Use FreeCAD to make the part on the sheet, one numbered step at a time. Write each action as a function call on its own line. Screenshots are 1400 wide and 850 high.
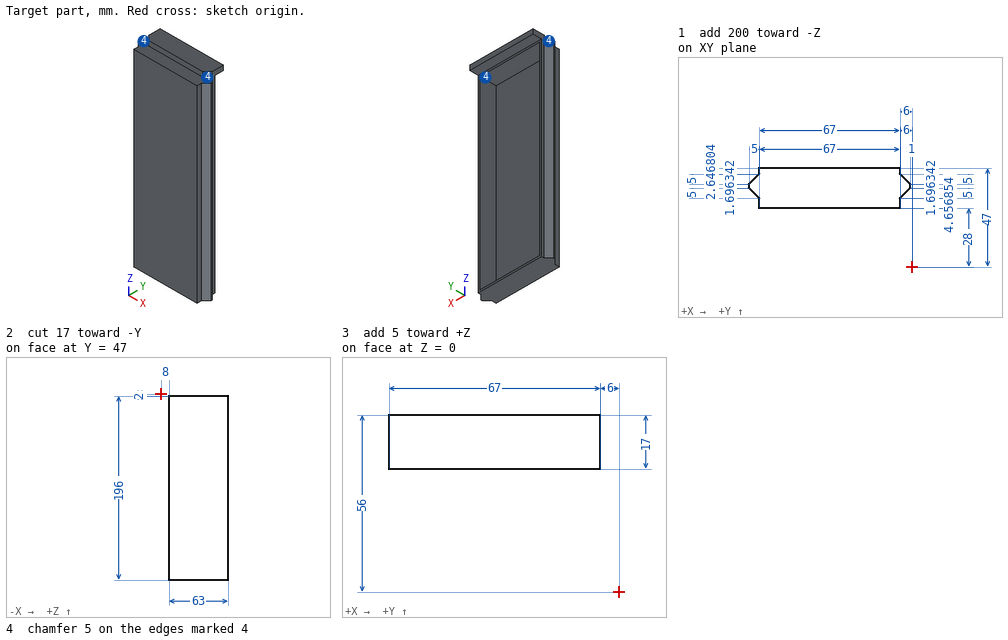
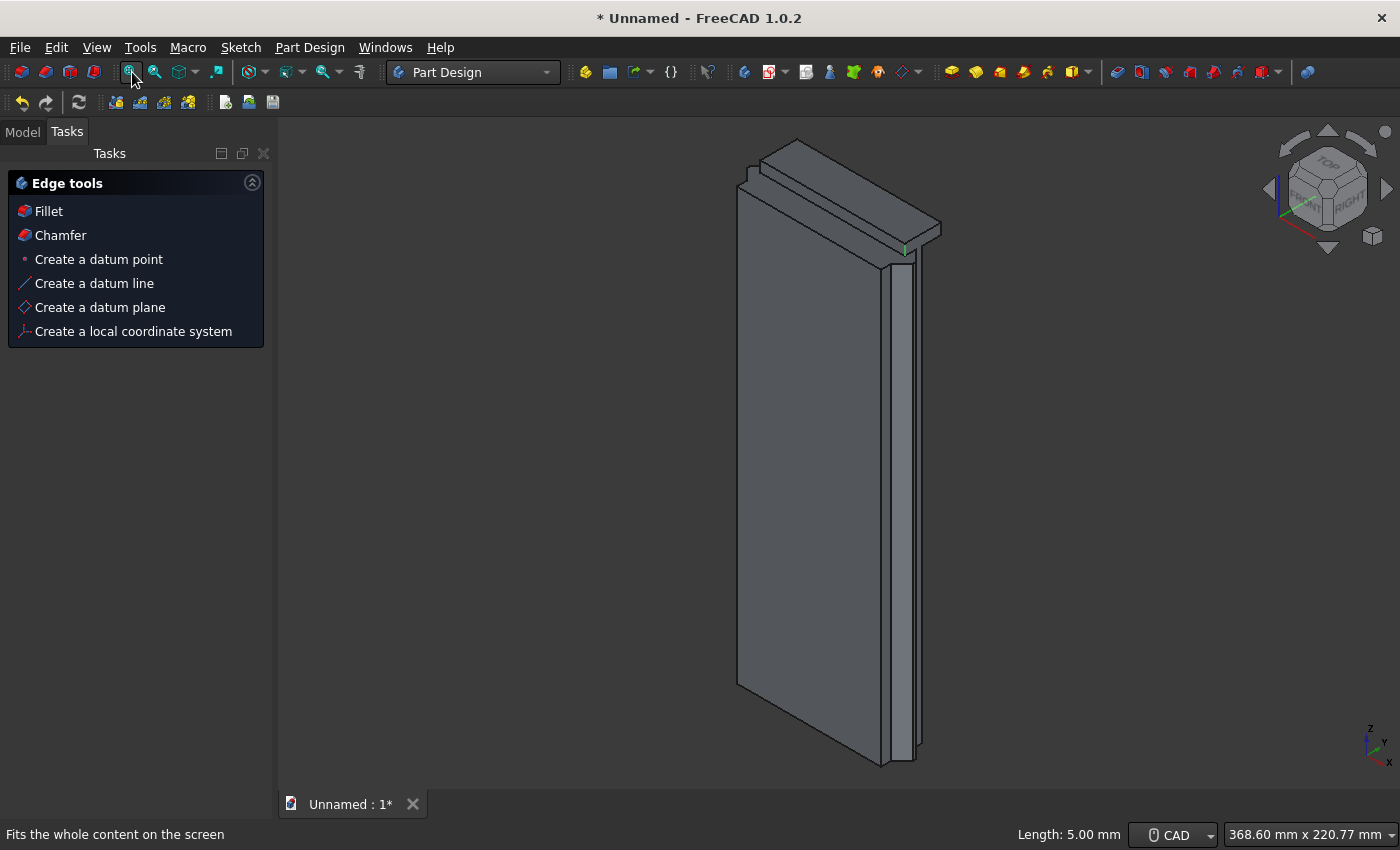
scroll(760, 166, up, 5)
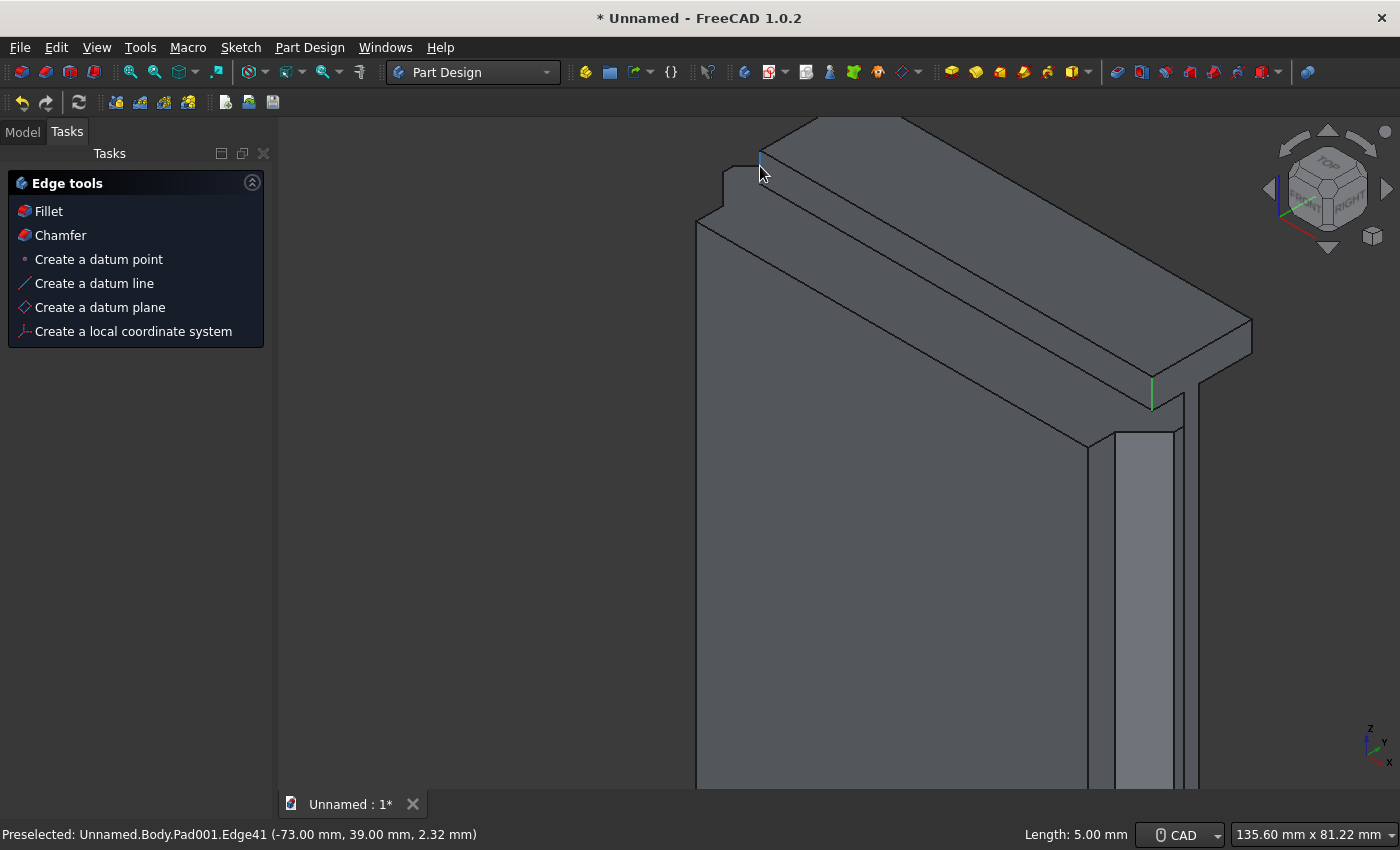
click(132, 72)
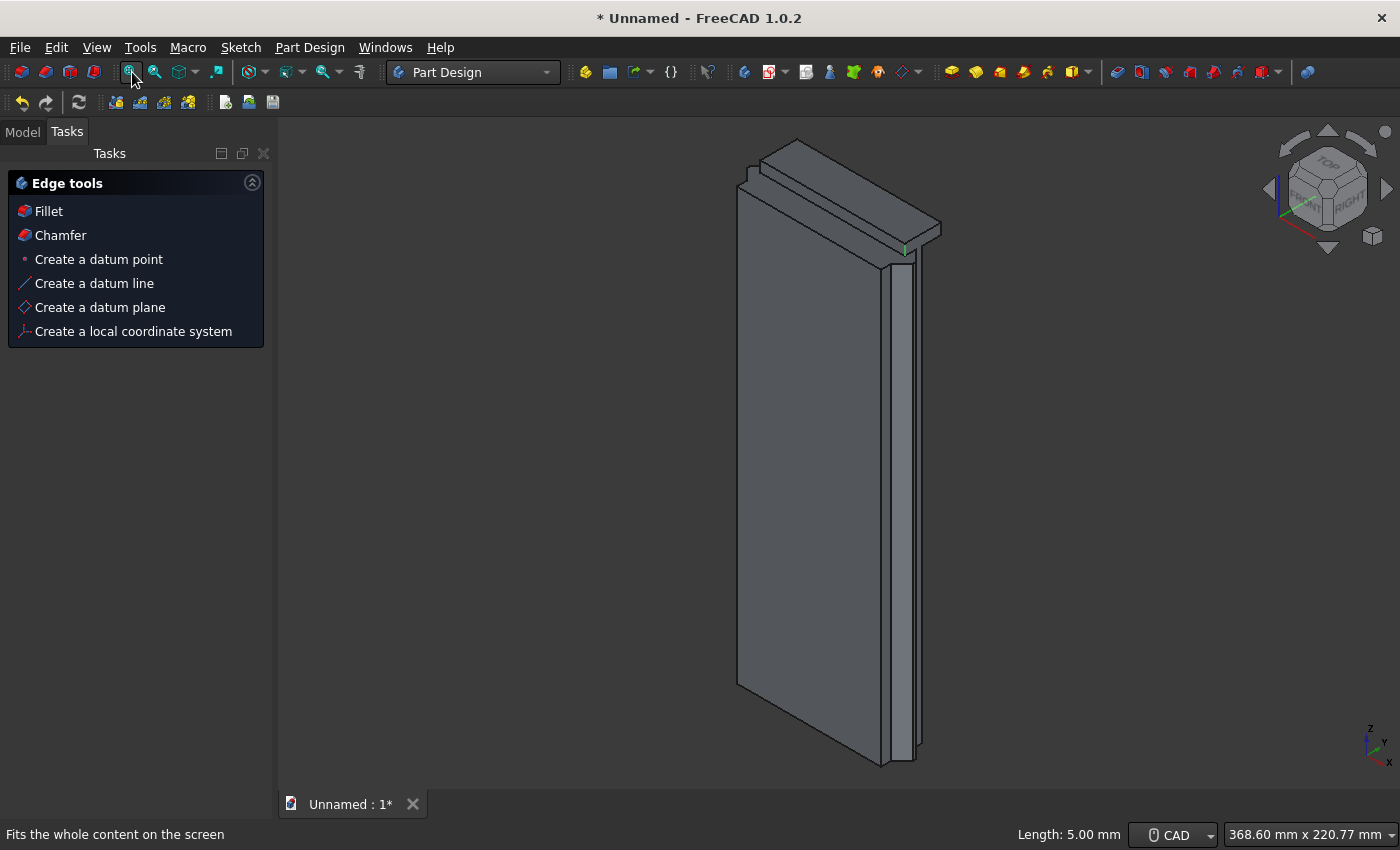
key(1)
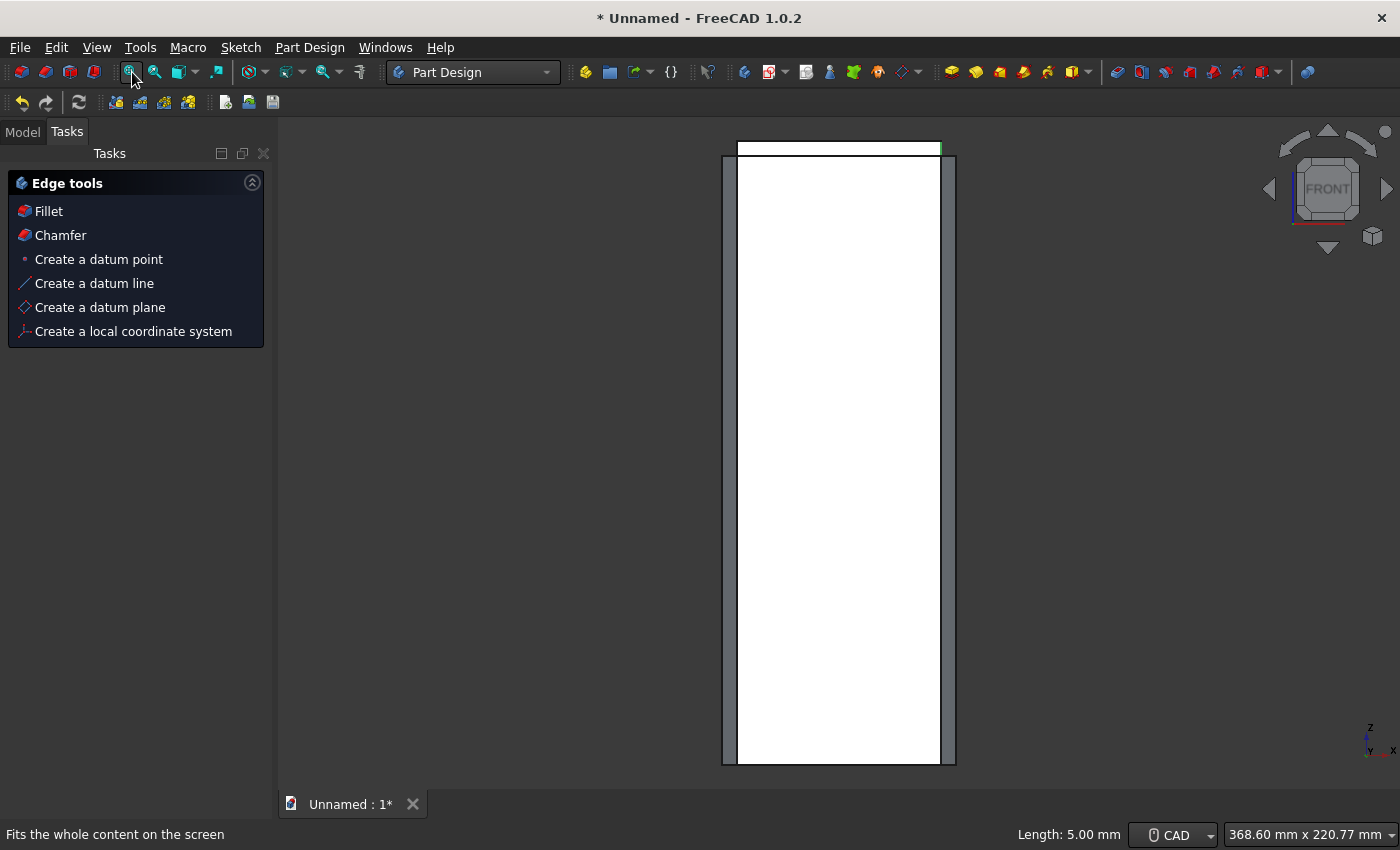
click(737, 148, ctrl)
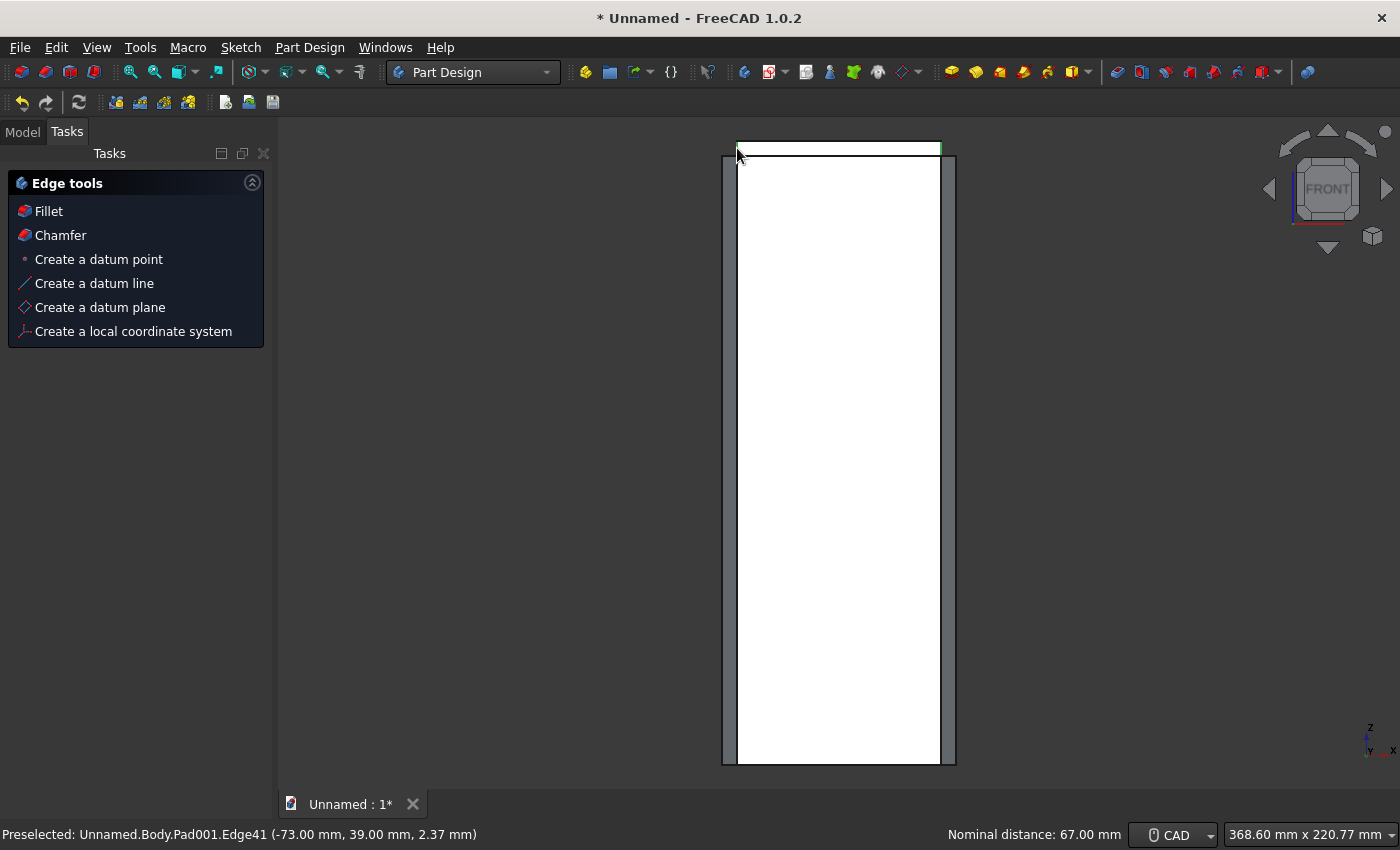
click(46, 72)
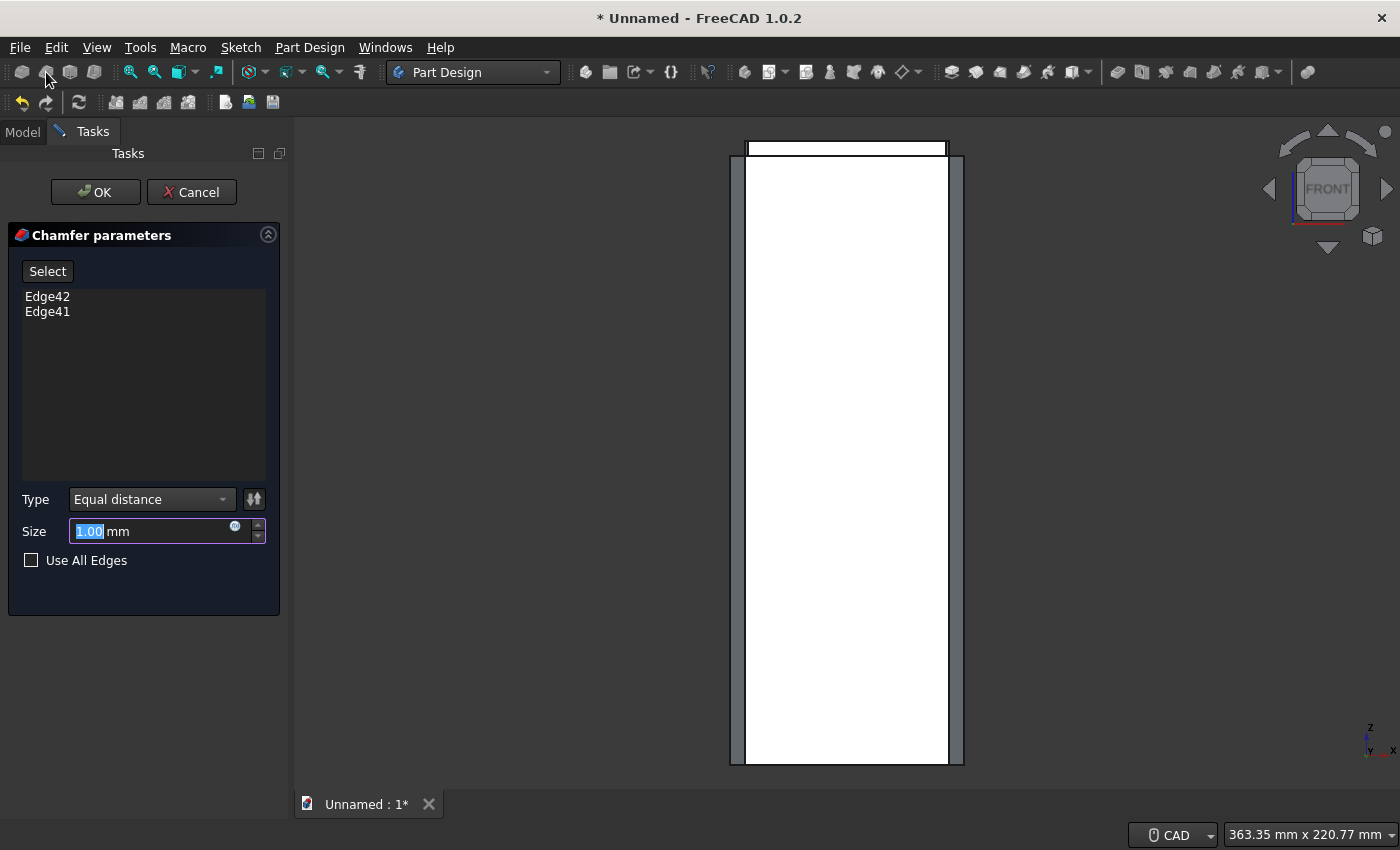
text(5)
key(Tab)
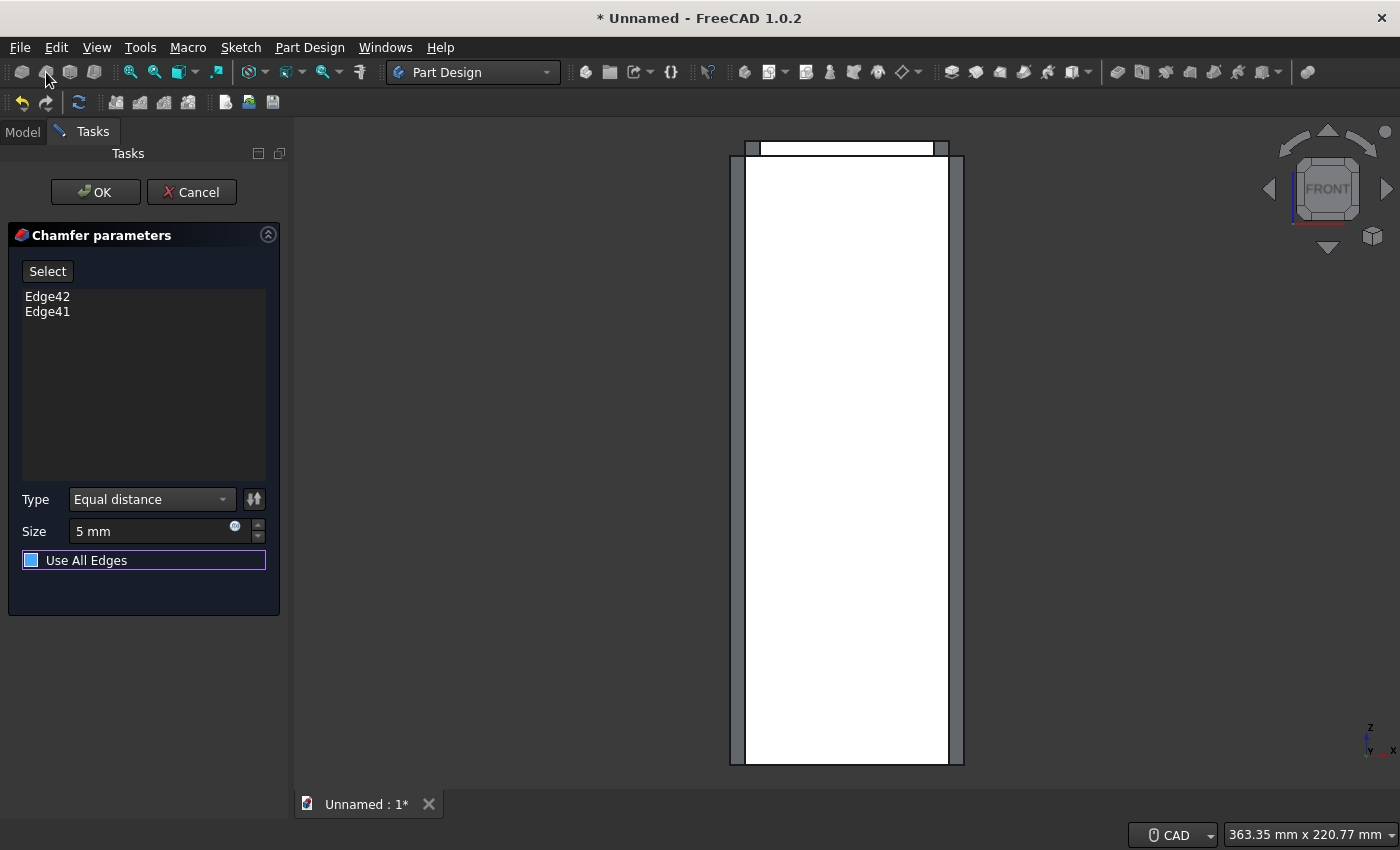
click(96, 192)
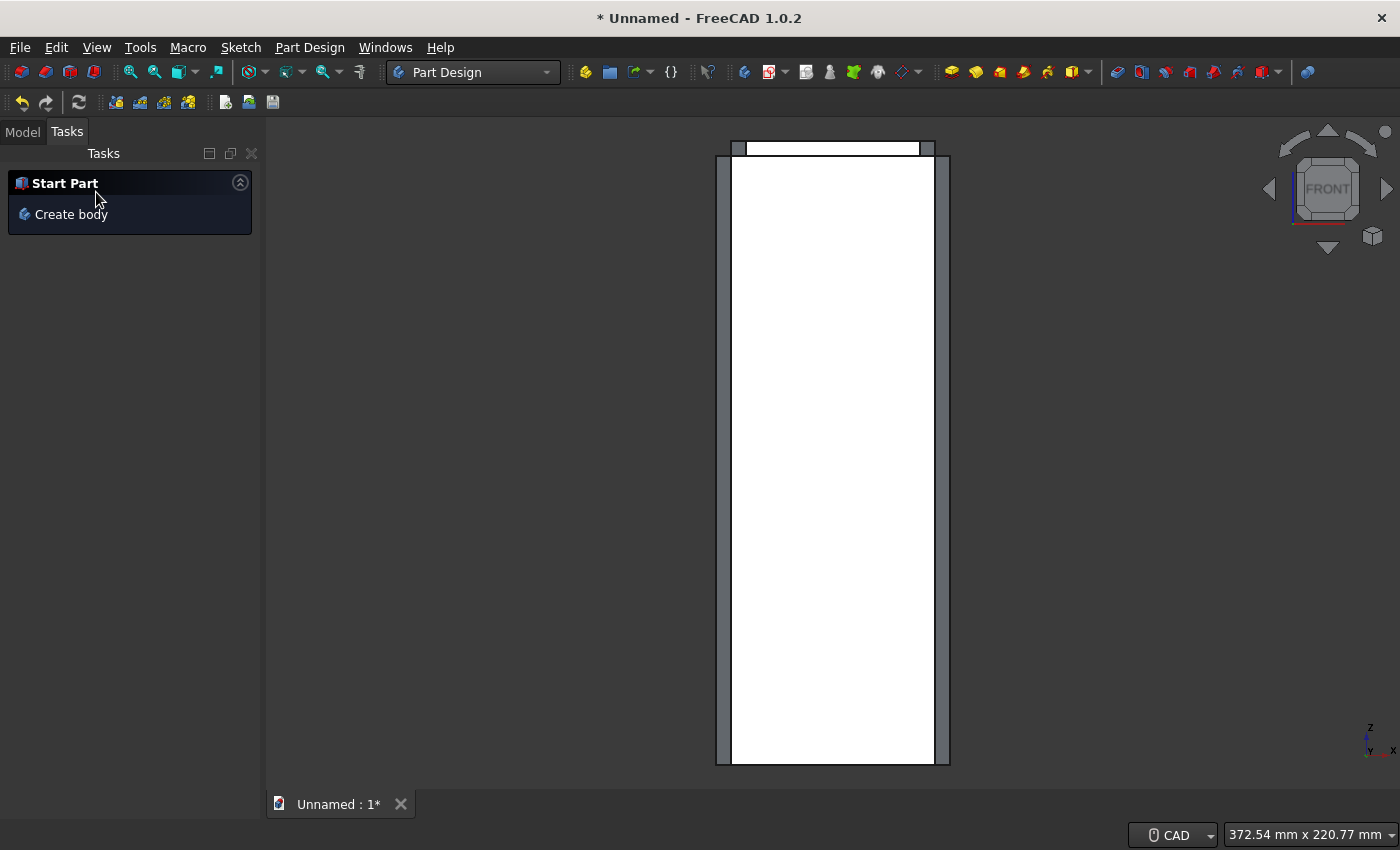
key(0)